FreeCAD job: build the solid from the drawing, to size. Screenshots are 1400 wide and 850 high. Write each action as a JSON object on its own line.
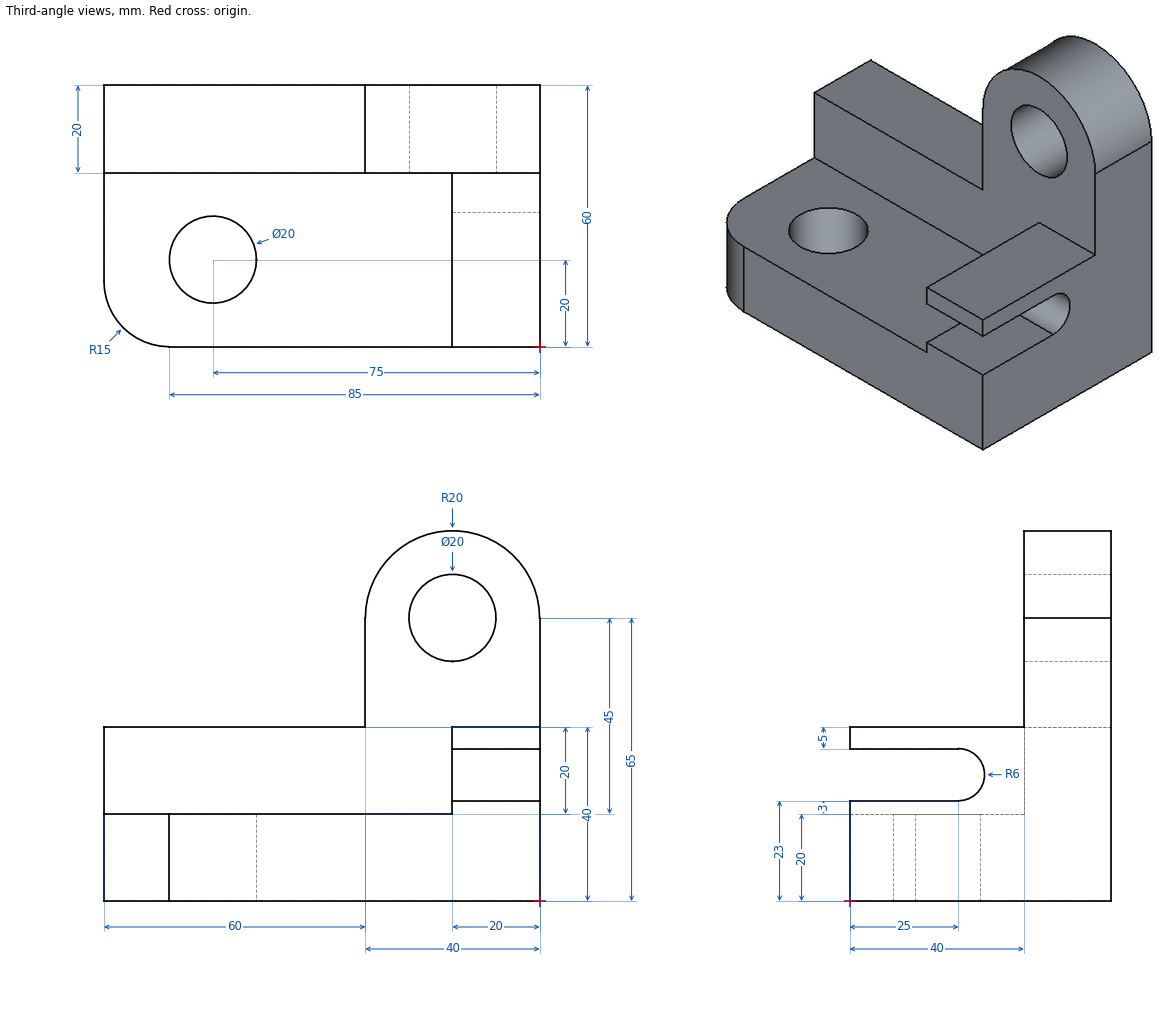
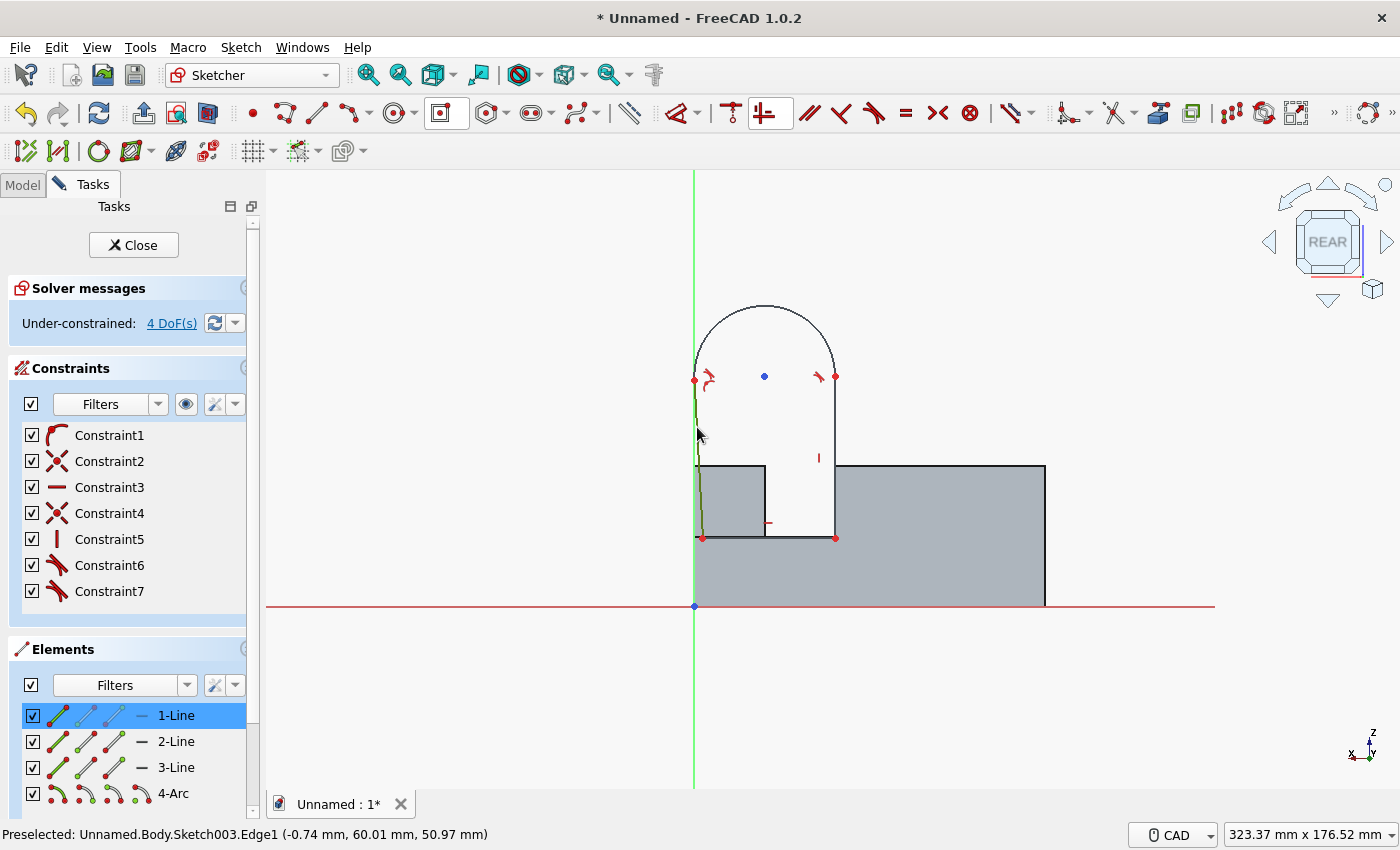
{"action": "key", "text": "v"}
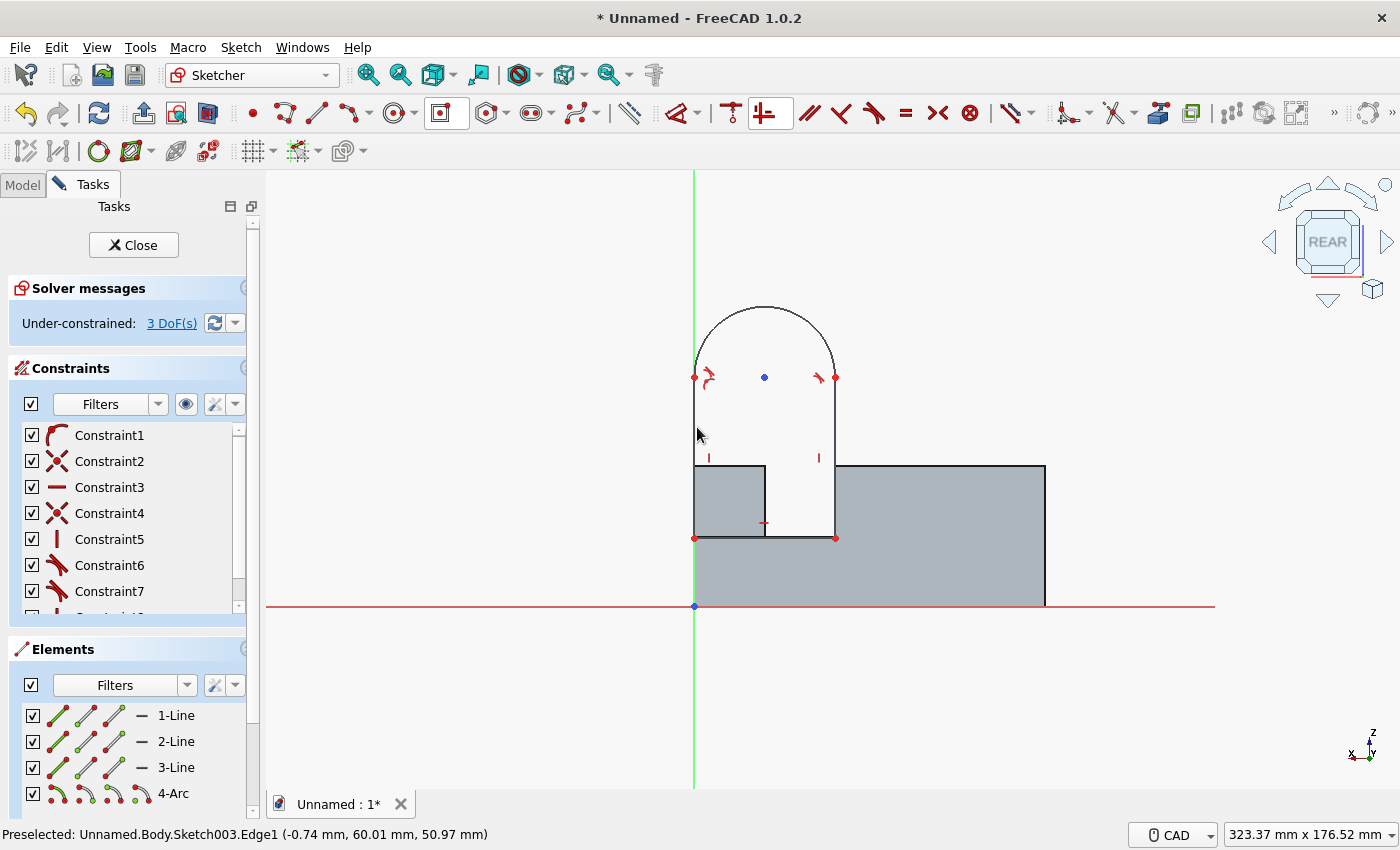
{"action": "key", "text": "d"}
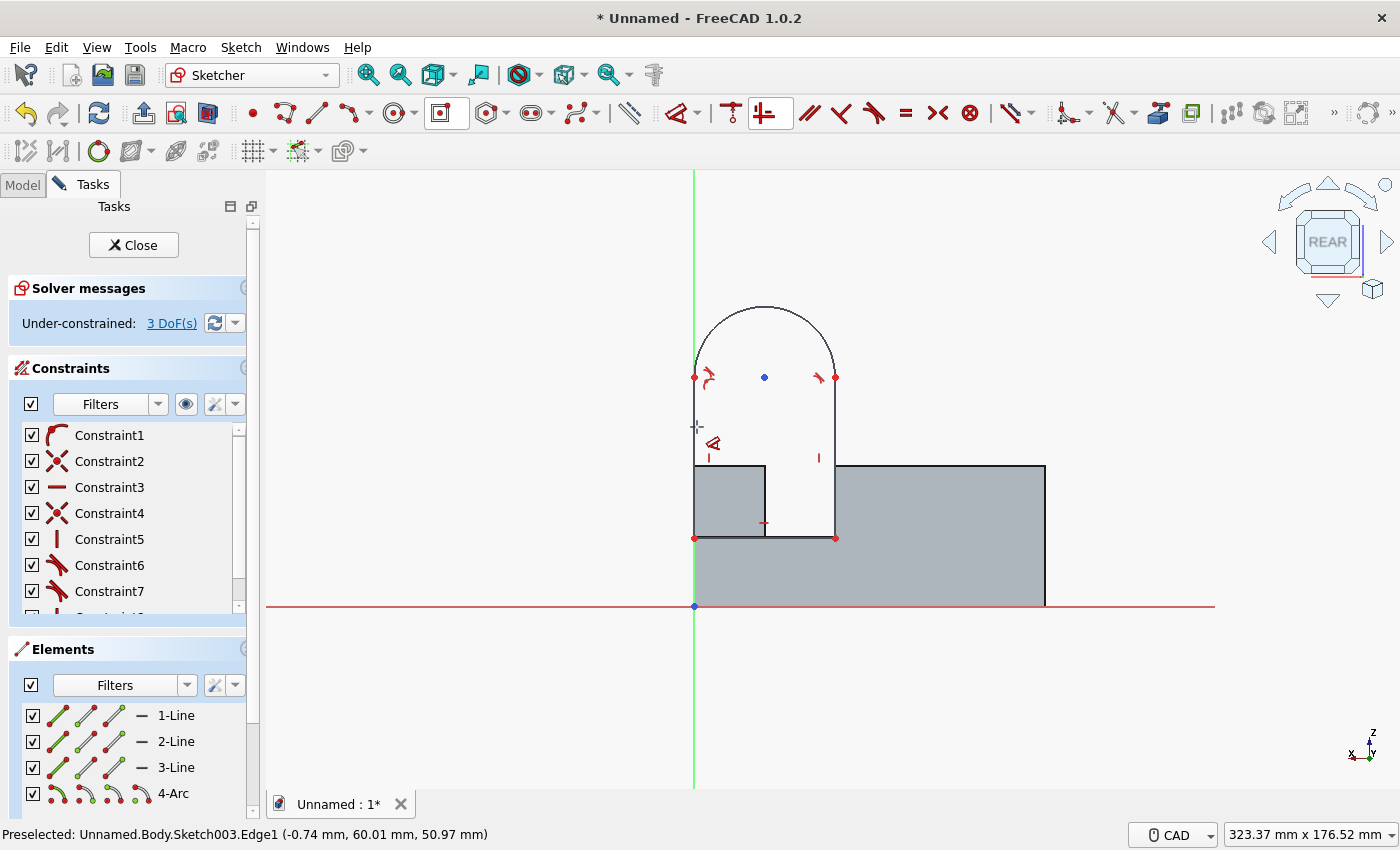
{"action": "left_click", "coordinate": [806, 320]}
{"action": "left_click", "coordinate": [825, 294]}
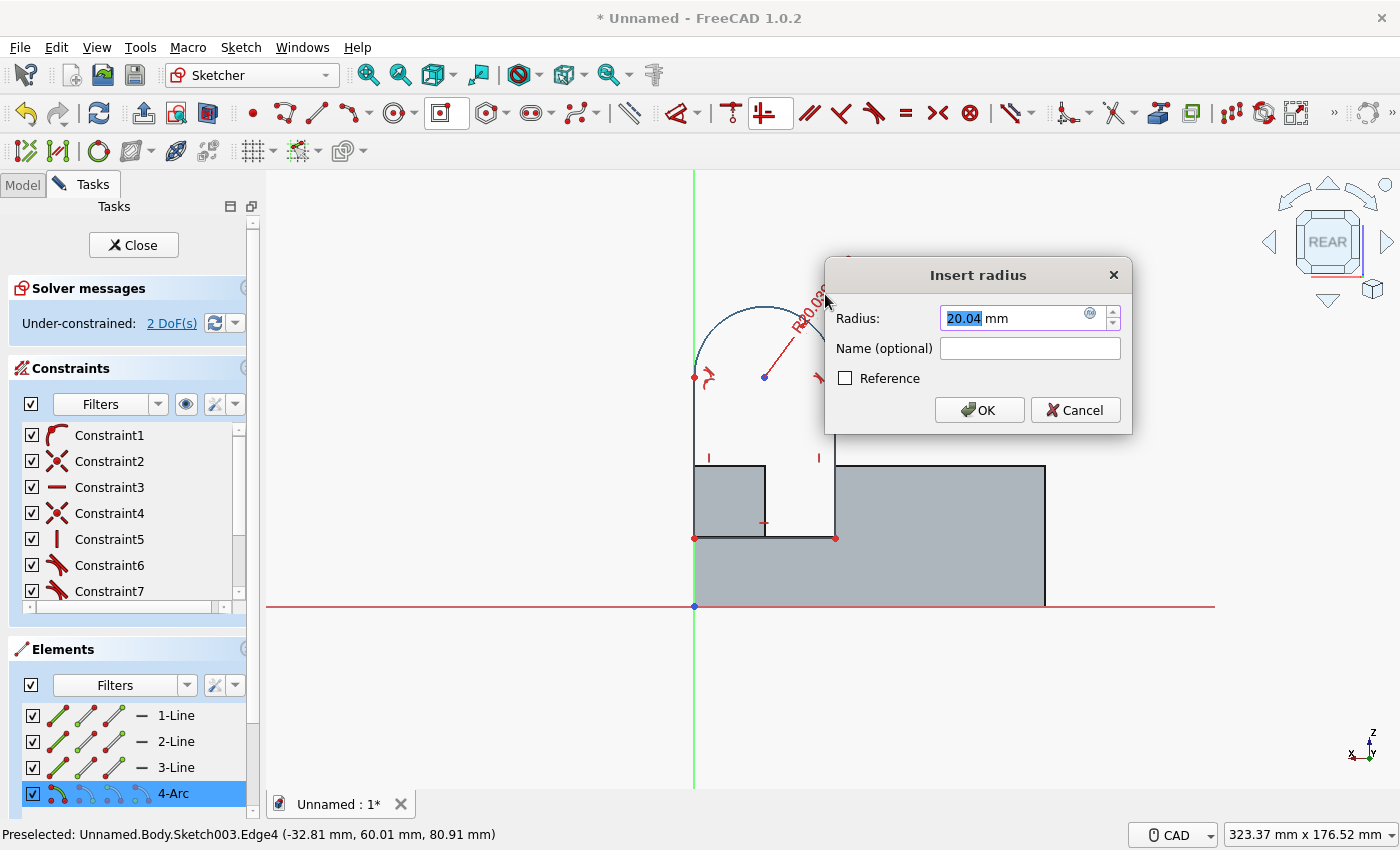
{"action": "type", "text": "20"}
{"action": "key", "text": "Return"}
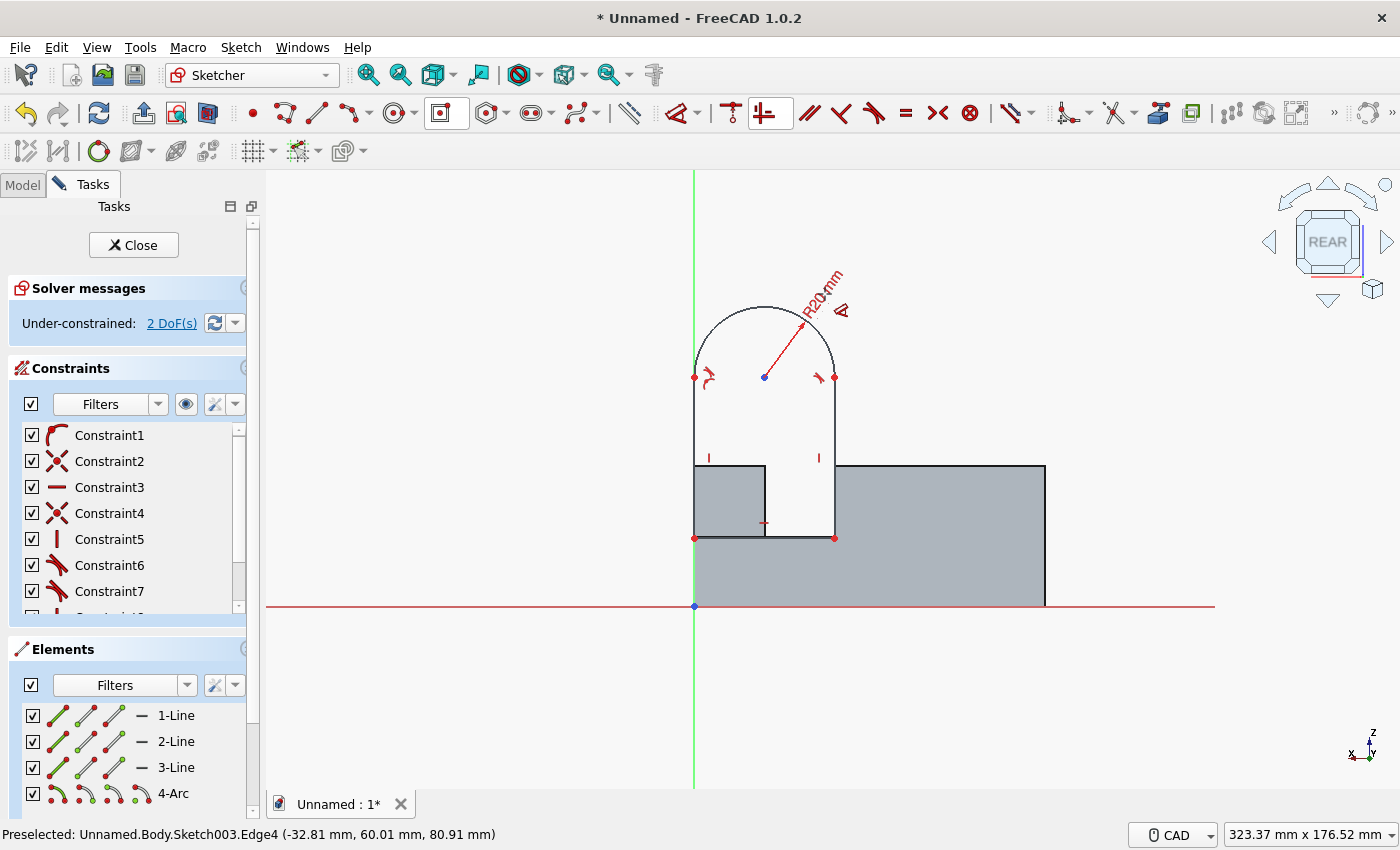
{"action": "left_click", "coordinate": [694, 425]}
{"action": "left_click", "coordinate": [660, 458]}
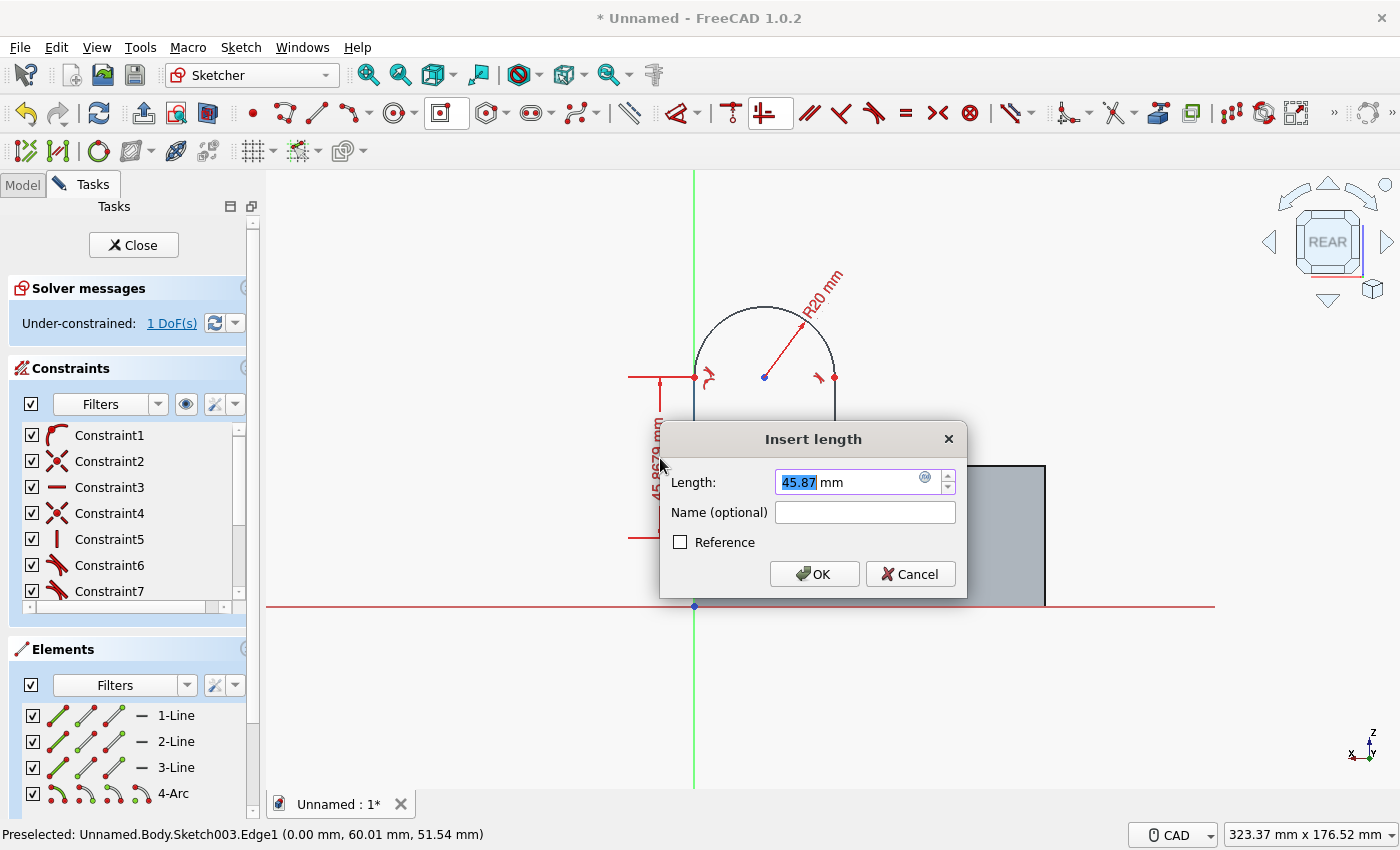
{"action": "type", "text": "45"}
{"action": "key", "text": "Return"}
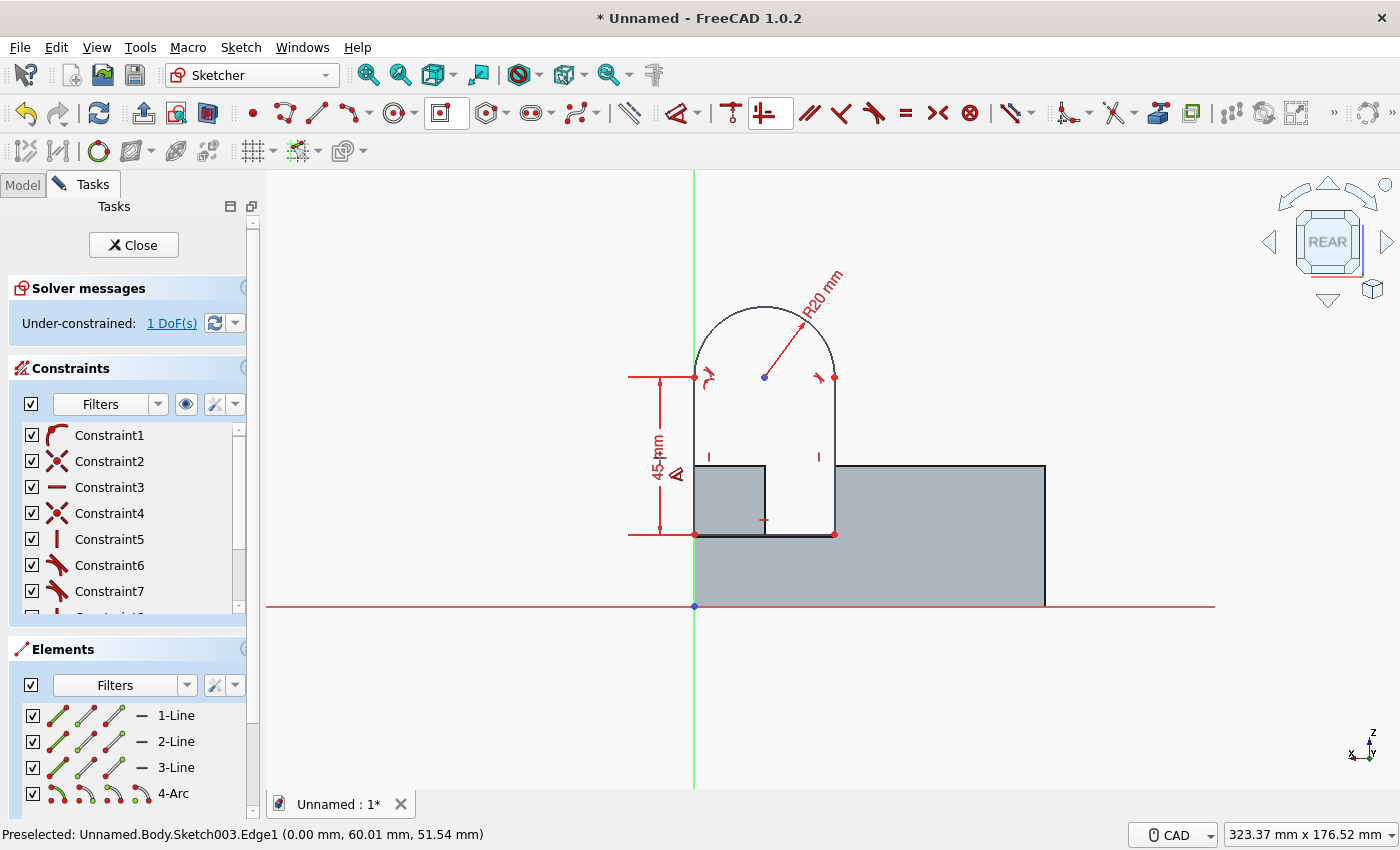
{"action": "left_click", "coordinate": [694, 377]}
{"action": "left_click", "coordinate": [660, 492]}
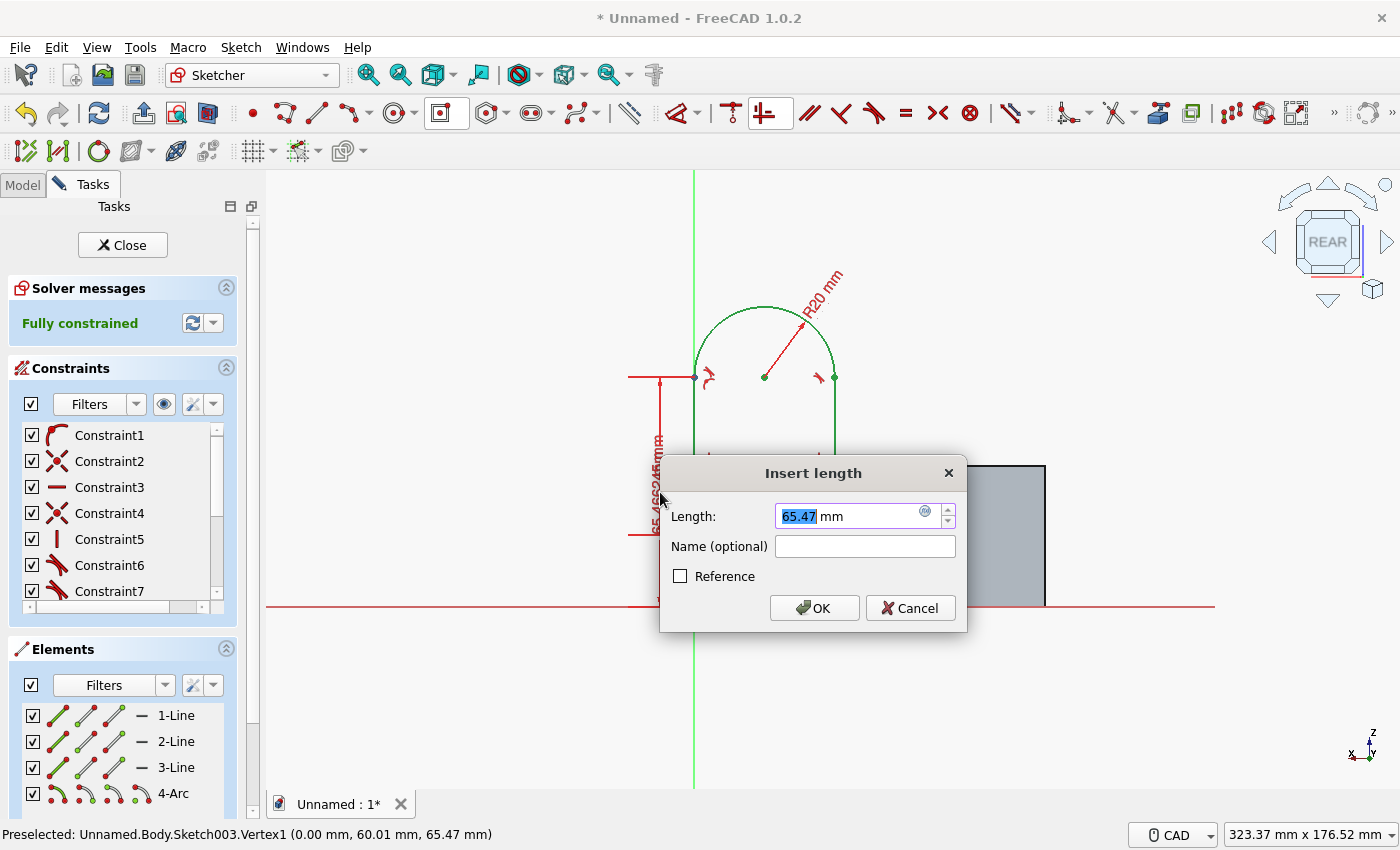
{"action": "type", "text": "65"}
{"action": "key", "text": "Return"}
{"action": "key", "text": "Escape"}